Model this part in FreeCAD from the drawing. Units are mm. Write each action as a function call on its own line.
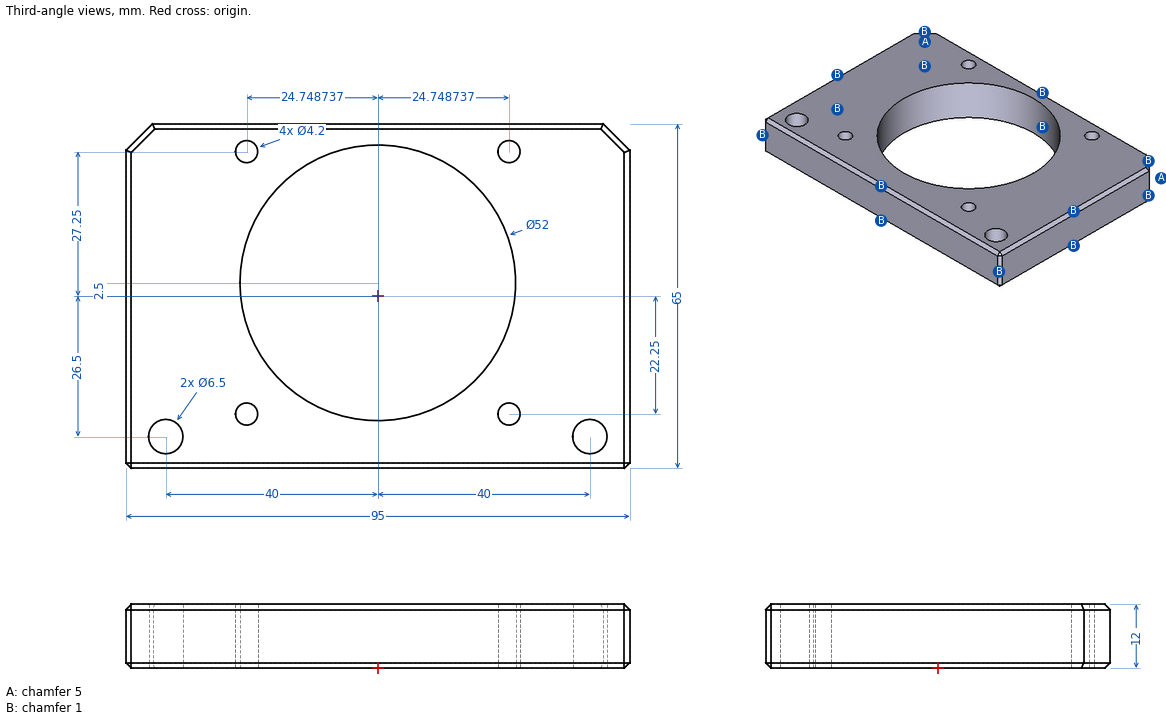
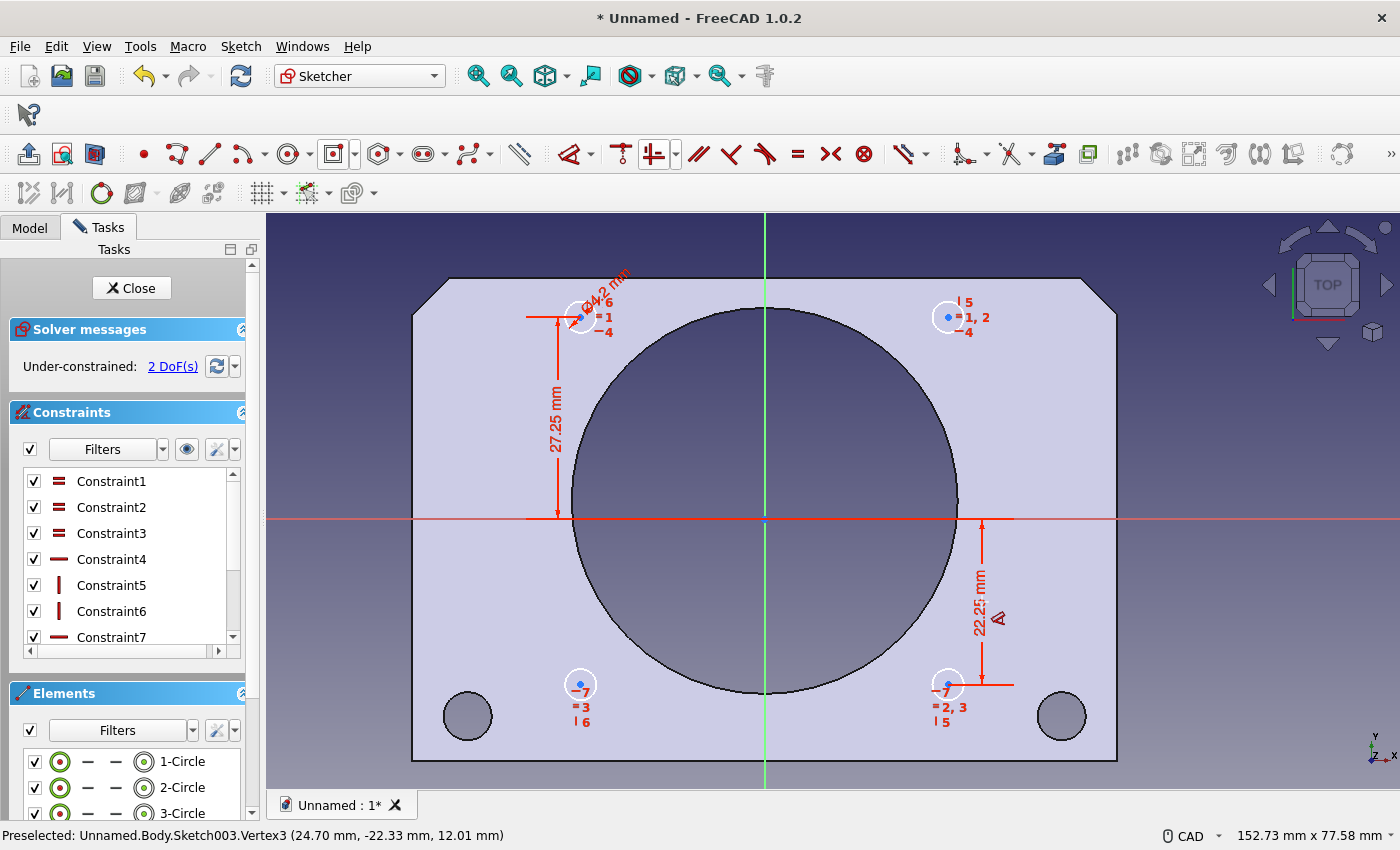
click(581, 317)
click(715, 283)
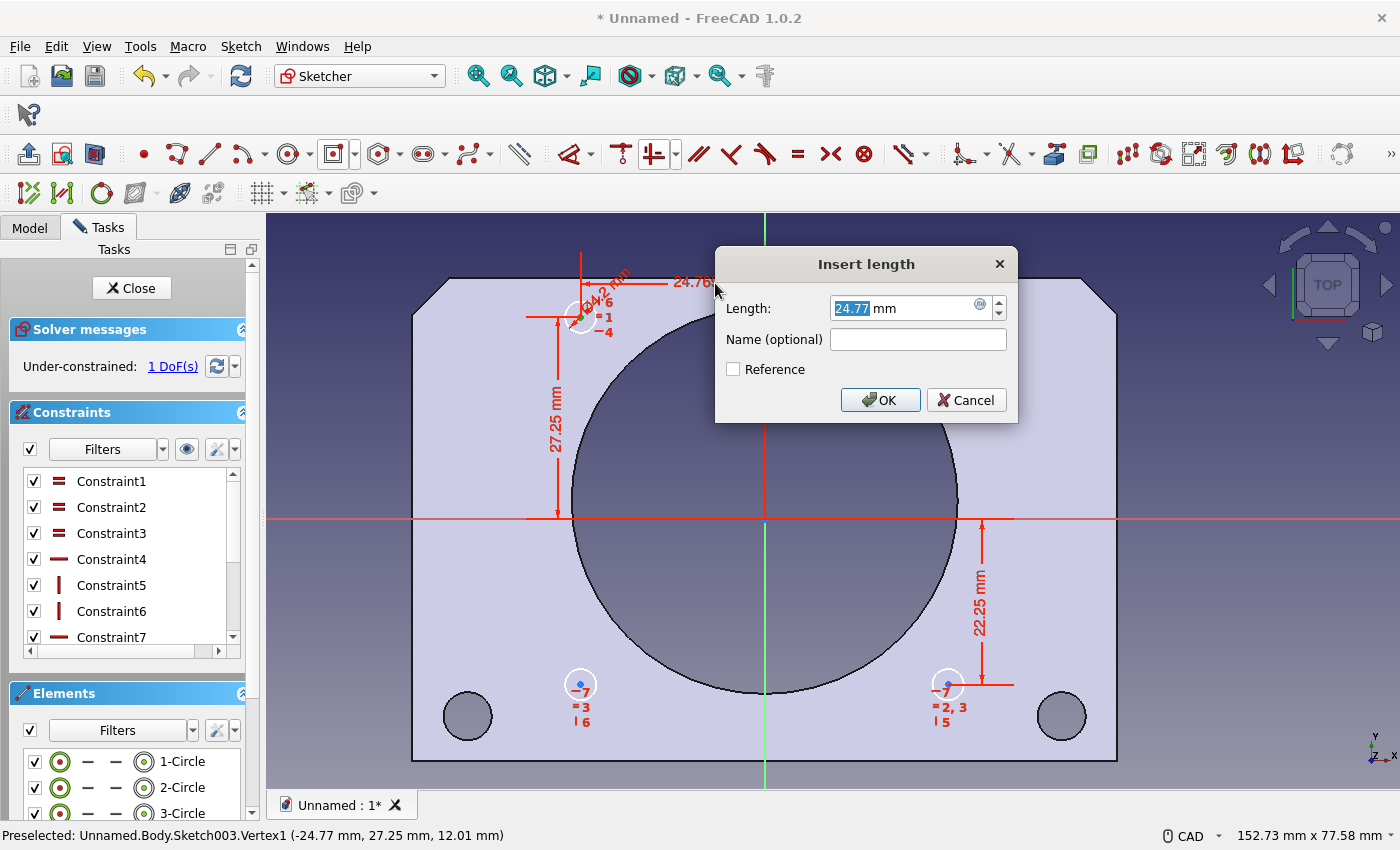
text(24.748737)
key(Return)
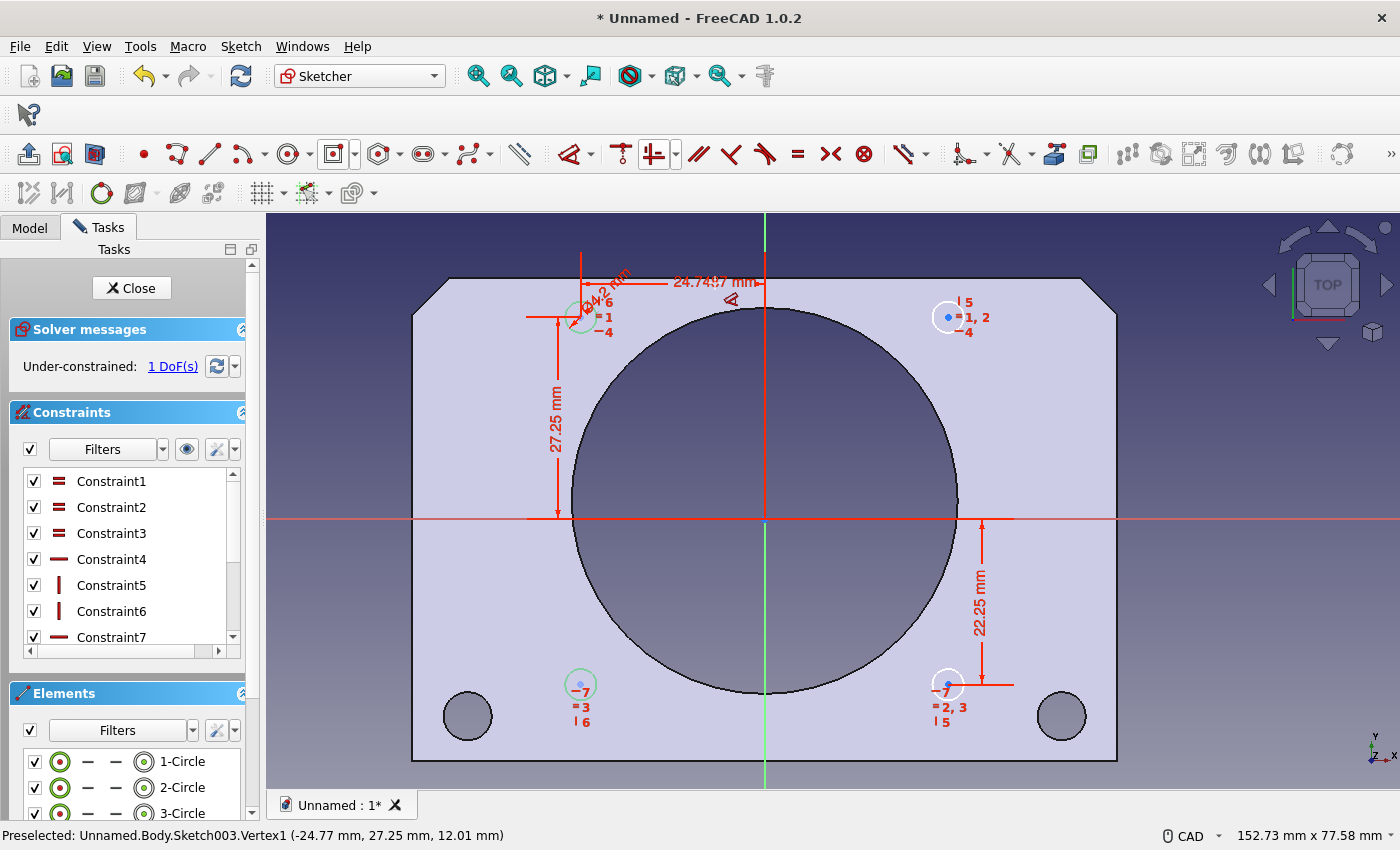
click(948, 317)
click(856, 283)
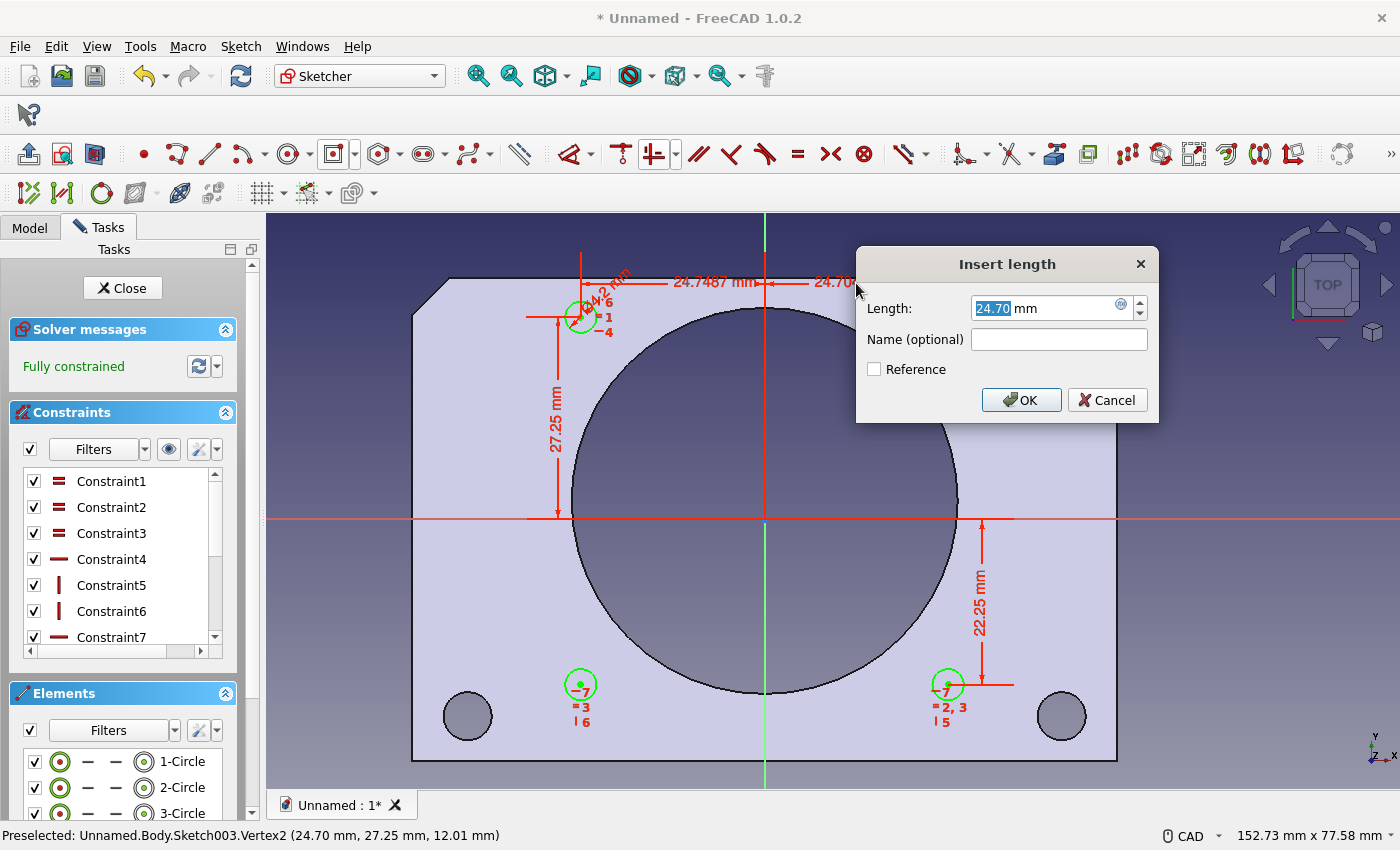
text(24.748737)
key(Return)
key(Escape)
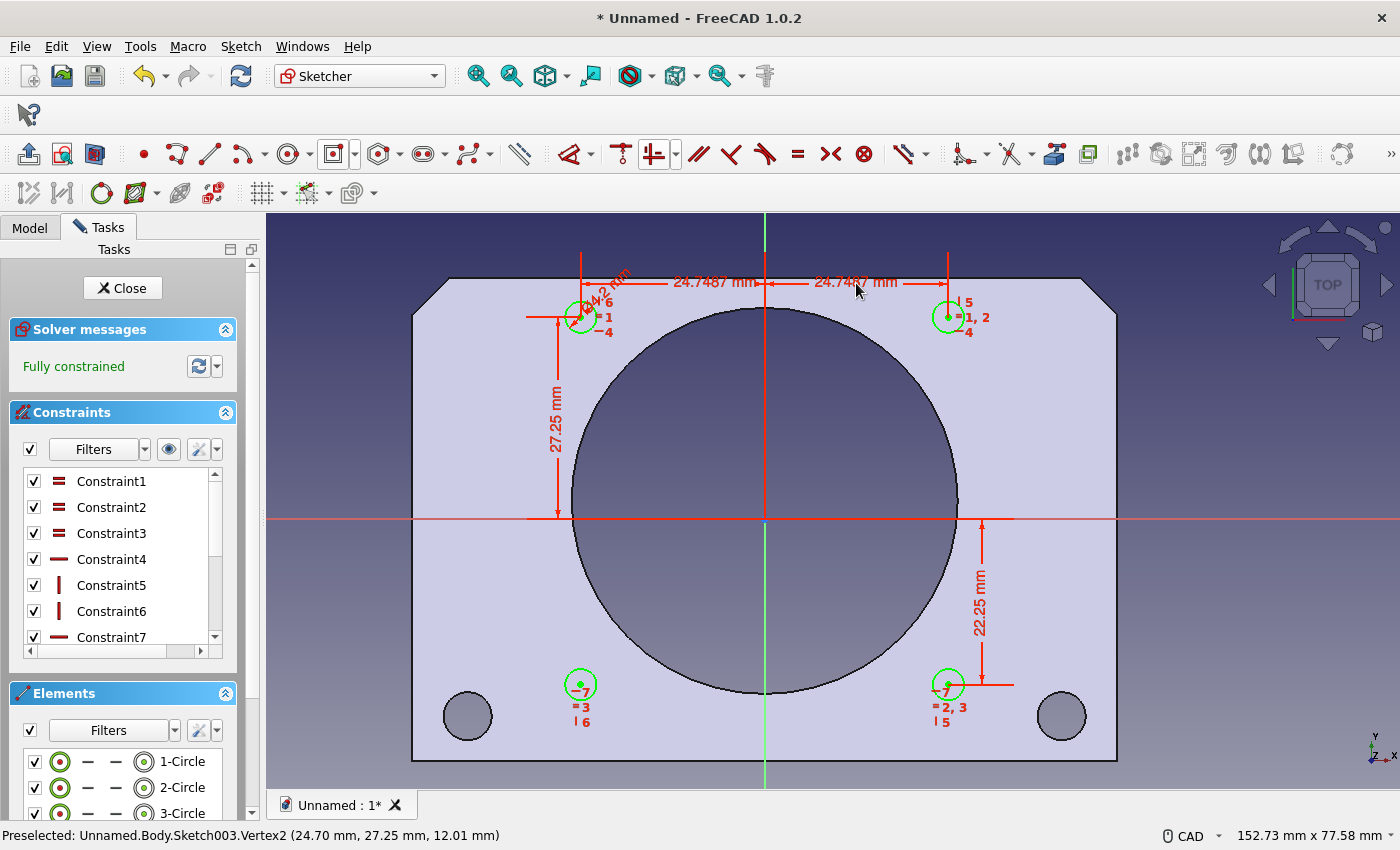
click(123, 288)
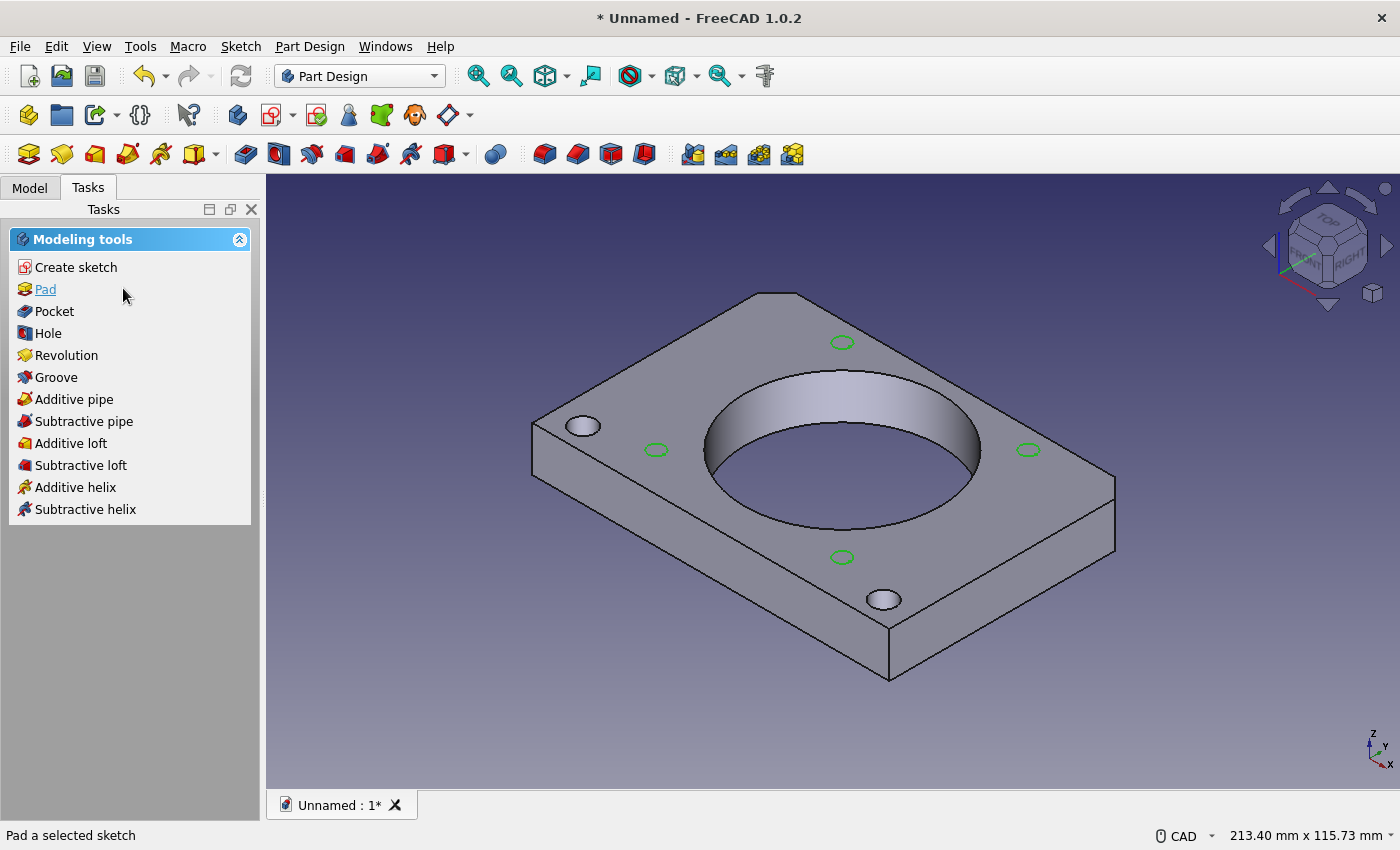
click(246, 154)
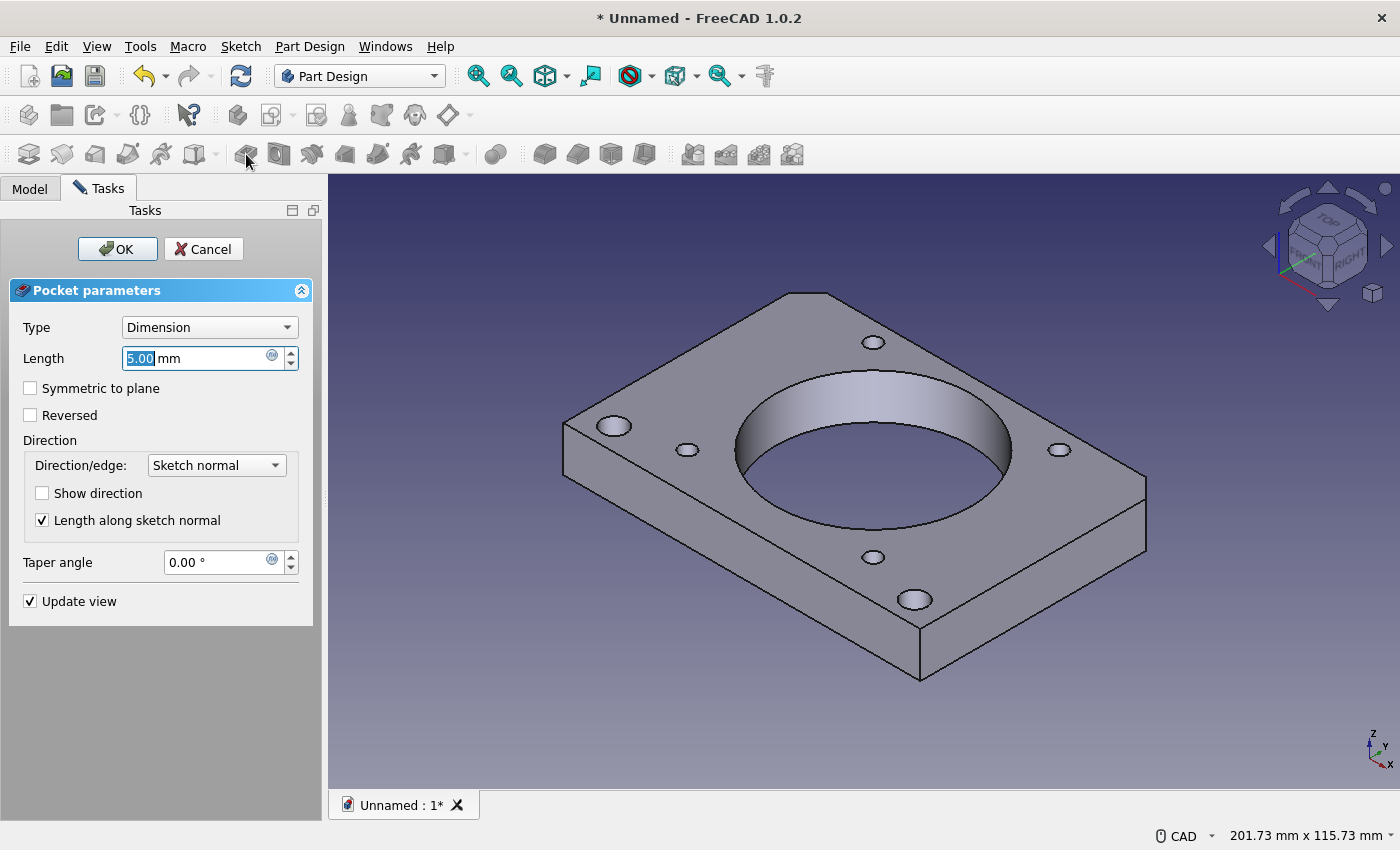
click(210, 328)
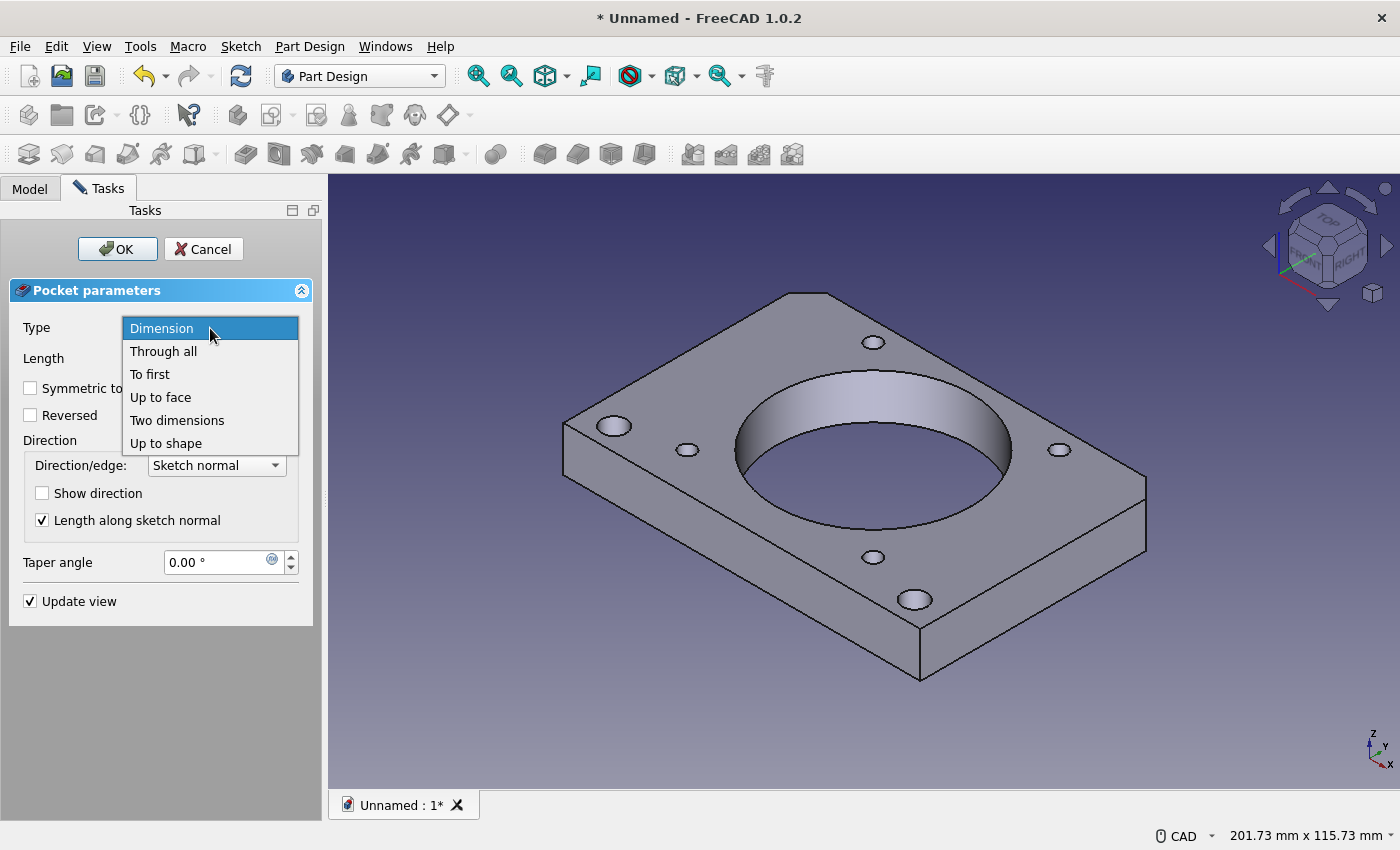
click(208, 352)